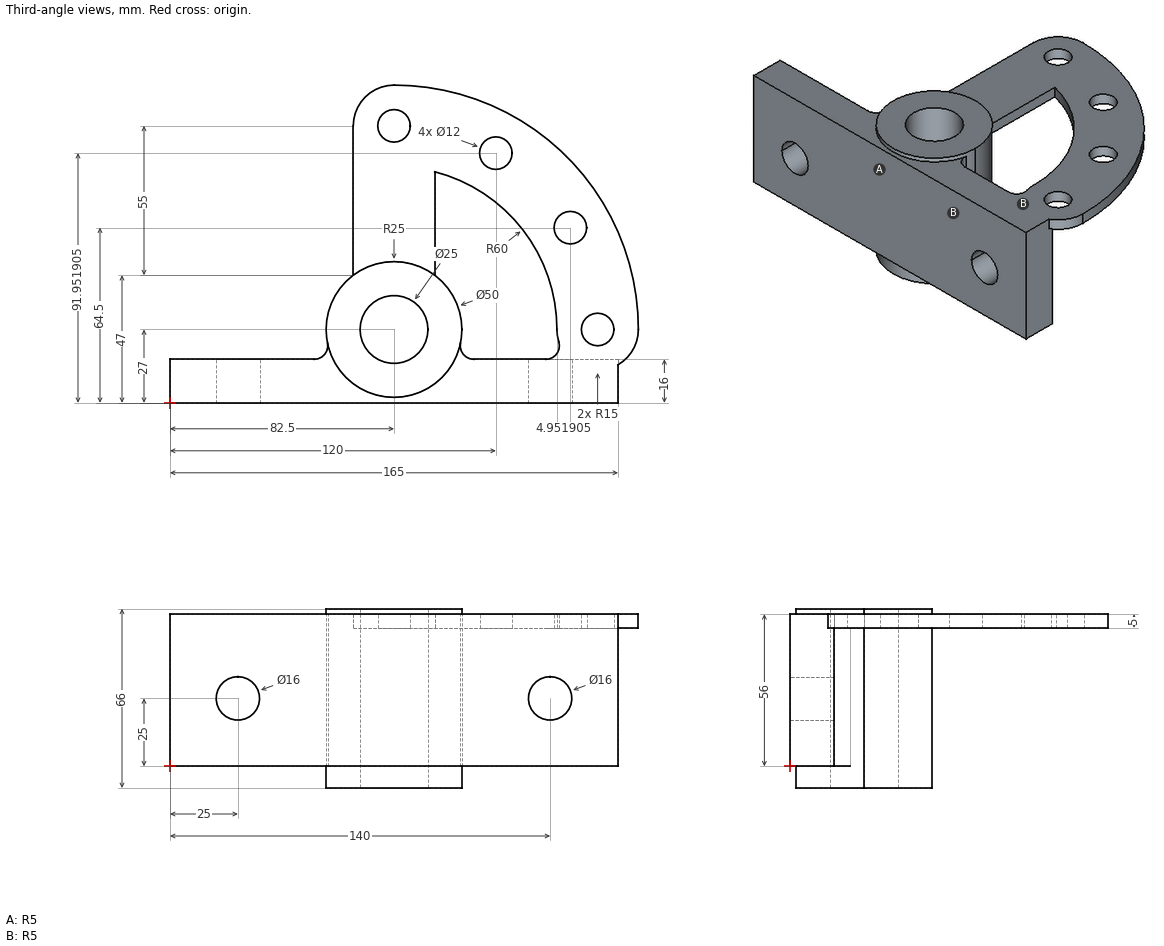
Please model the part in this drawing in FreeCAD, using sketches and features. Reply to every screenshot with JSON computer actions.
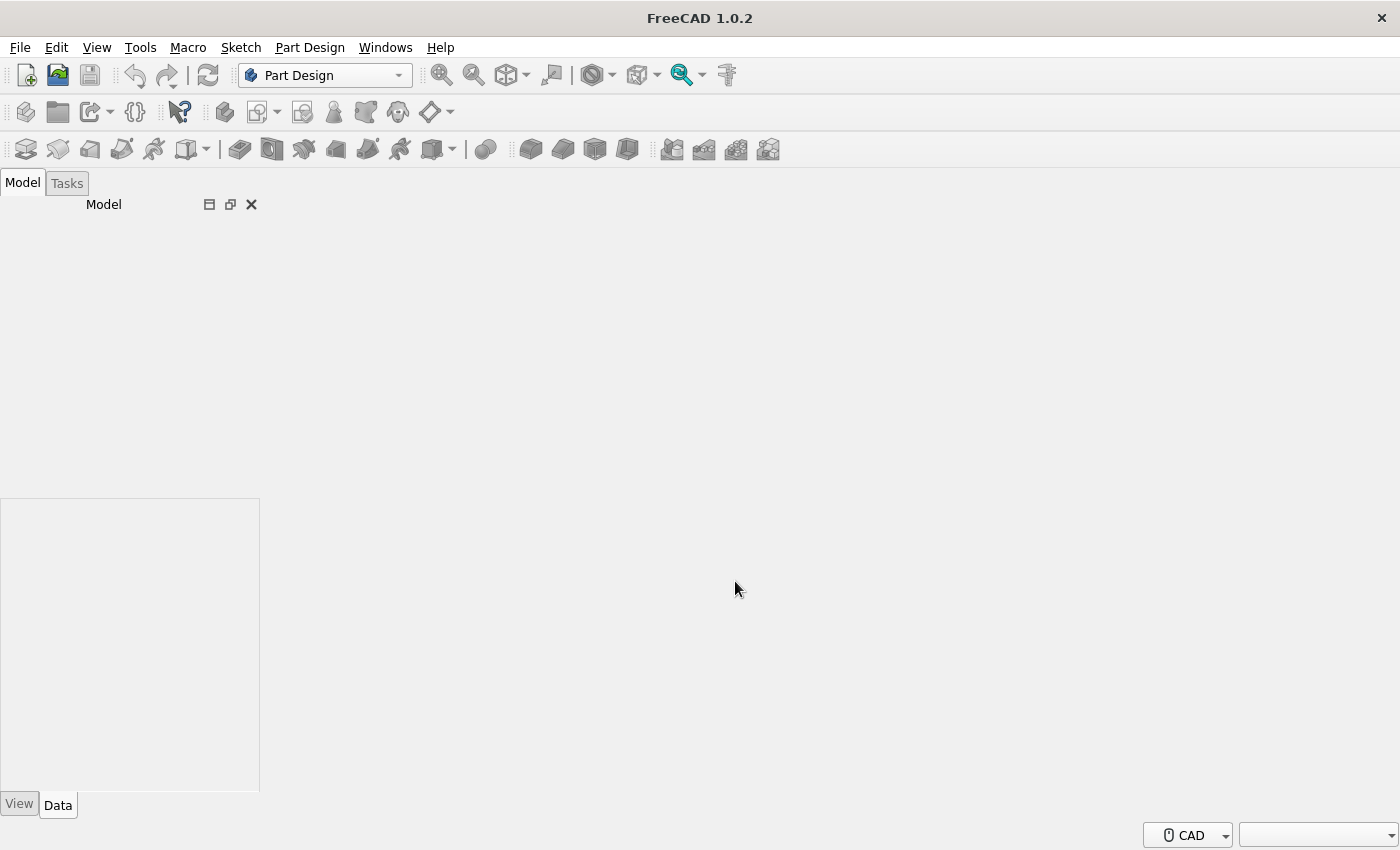
{"action": "left_click", "coordinate": [26, 76]}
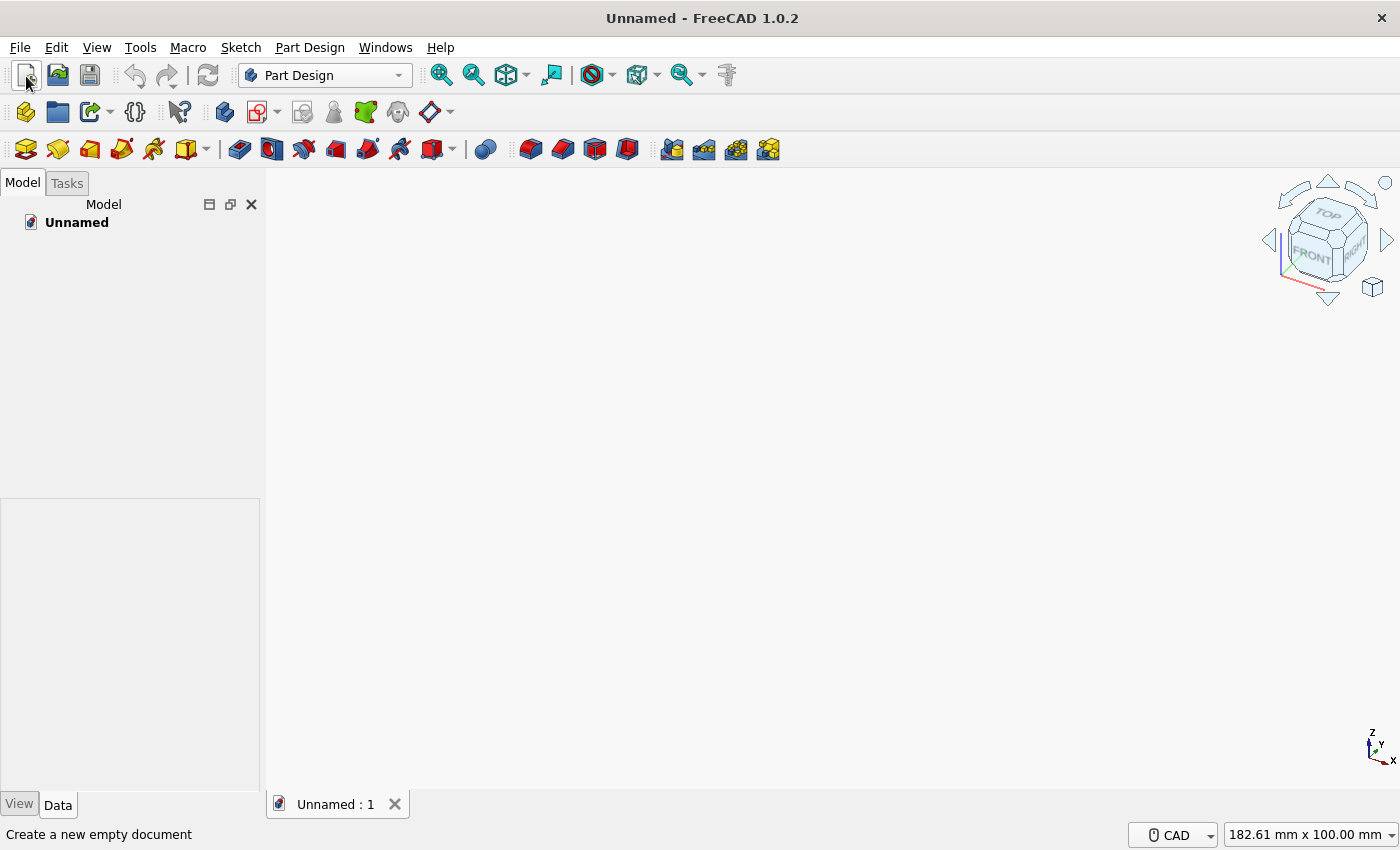
{"action": "left_click", "coordinate": [258, 112]}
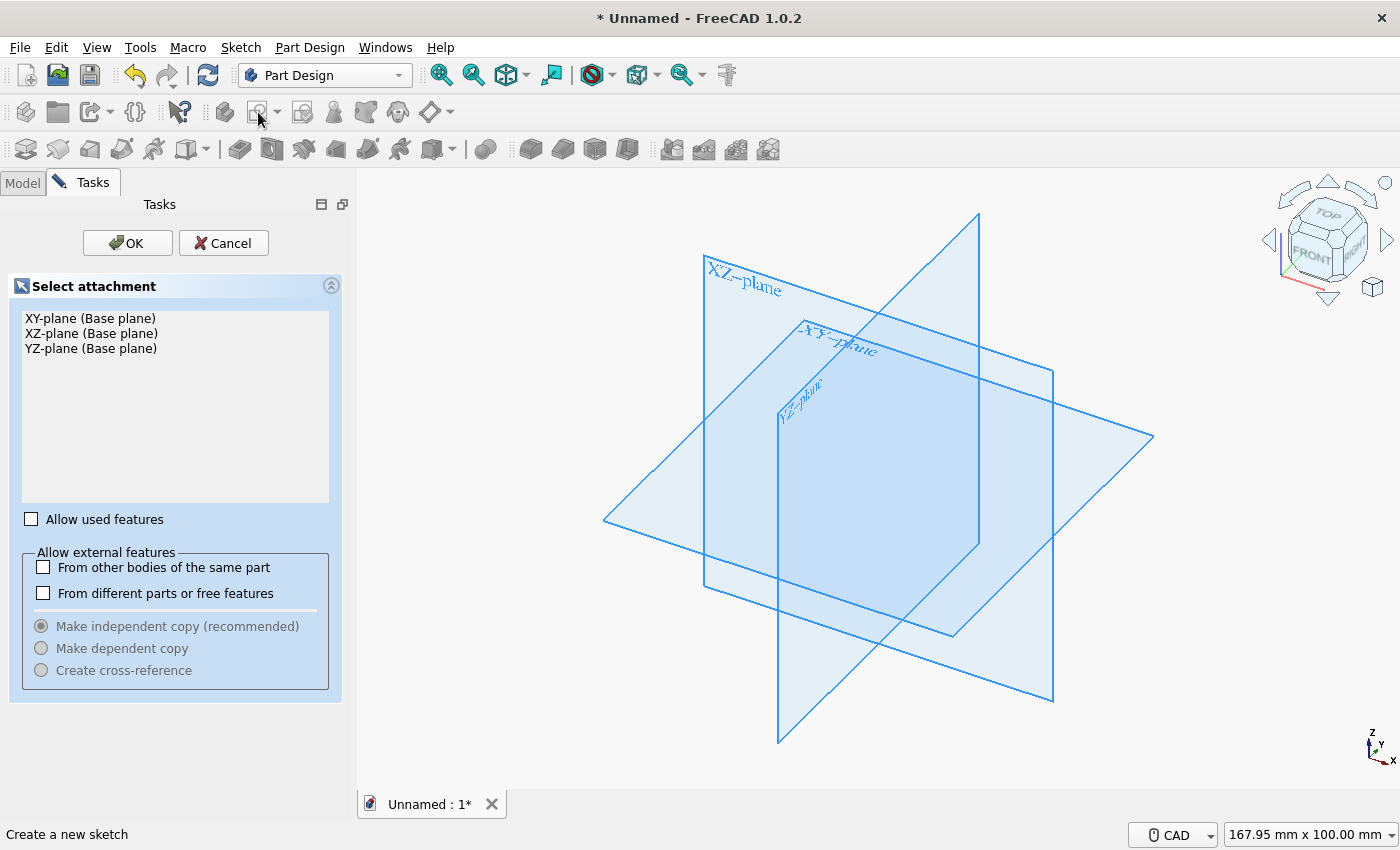
{"action": "left_click", "coordinate": [82, 318]}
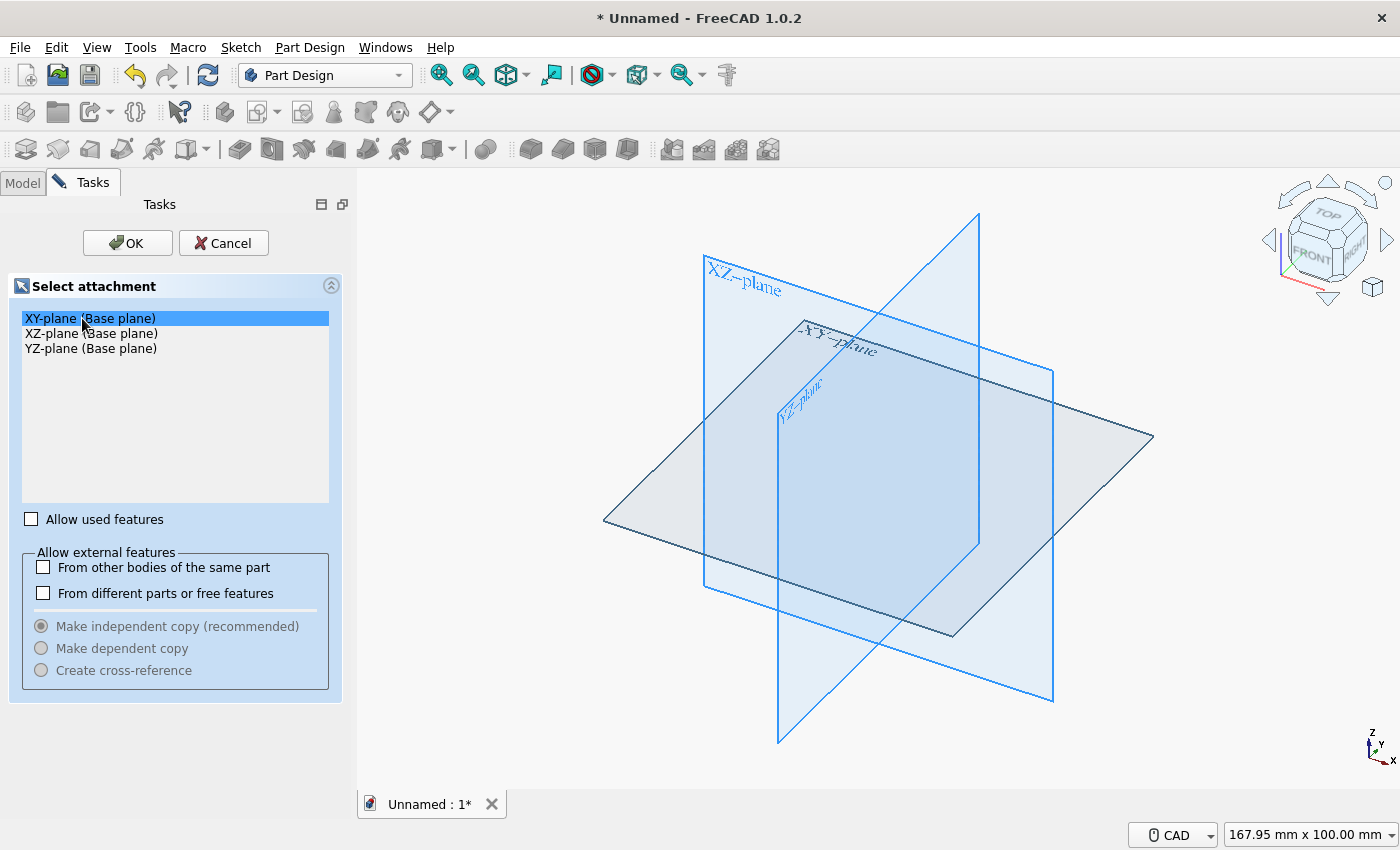
{"action": "left_click", "coordinate": [128, 243]}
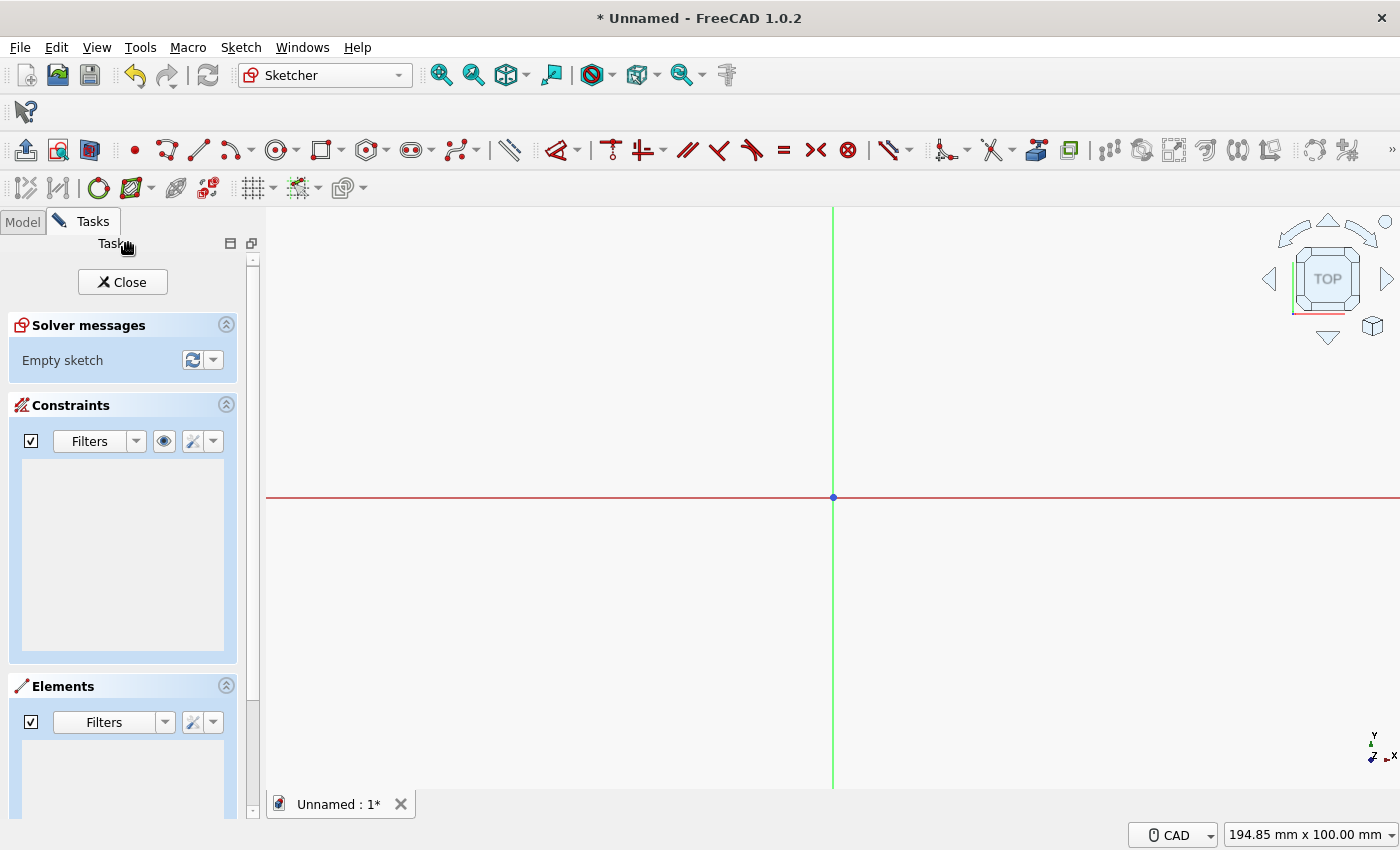
{"action": "scroll", "coordinate": [294, 555], "scroll_direction": "down", "scroll_amount": 3}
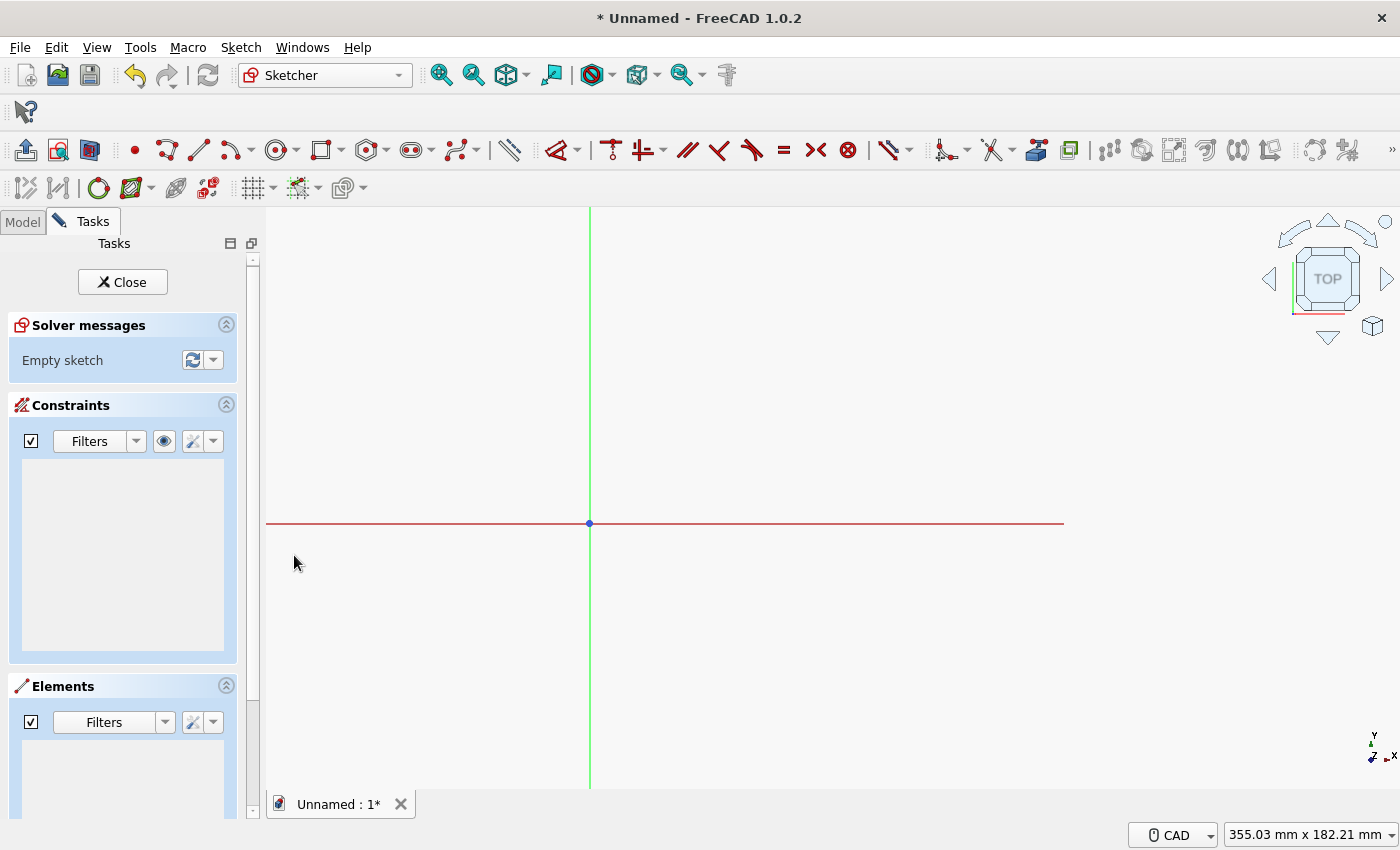
{"action": "left_click", "coordinate": [322, 150]}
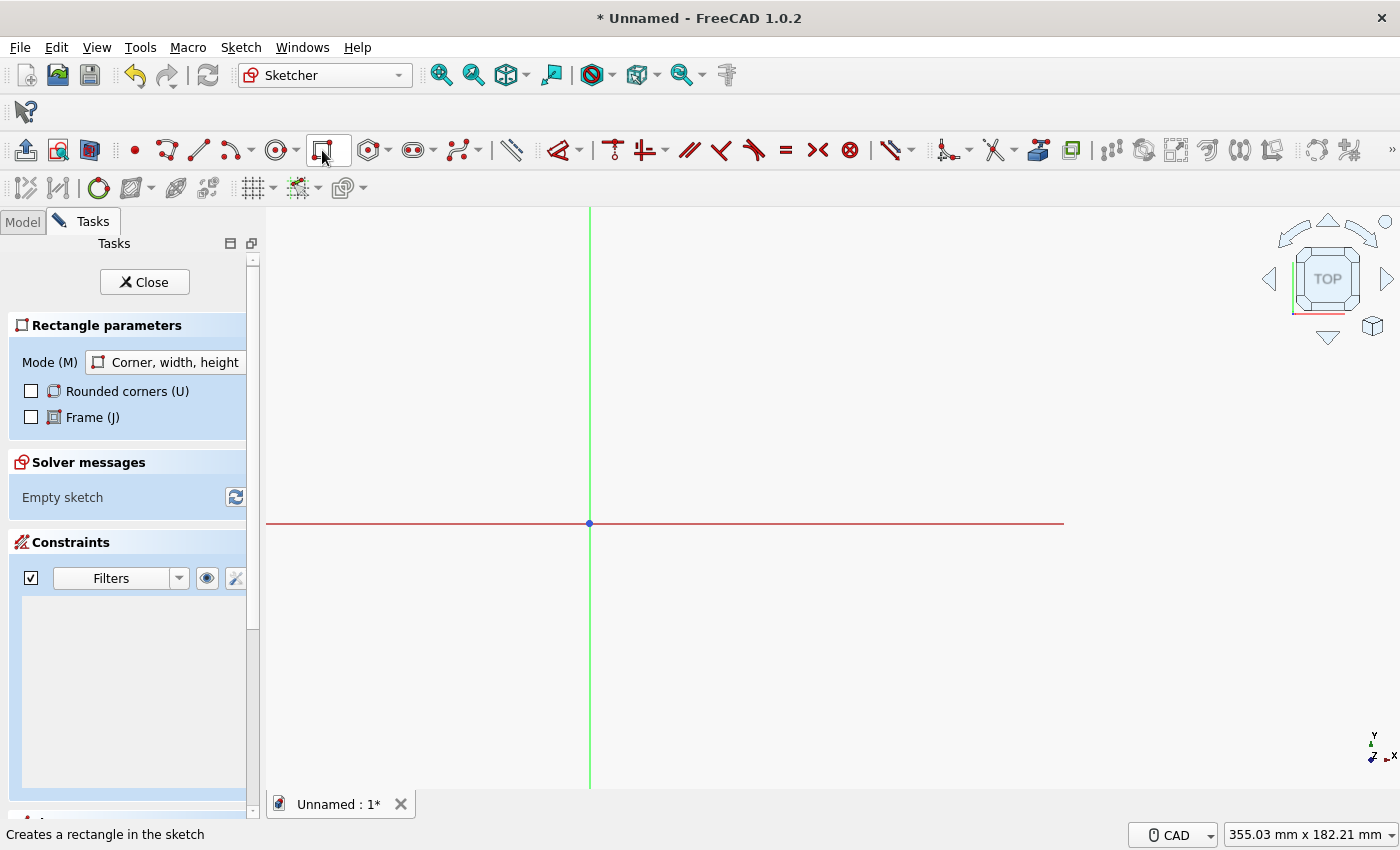
{"action": "left_click", "coordinate": [590, 524]}
{"action": "left_click", "coordinate": [1117, 473]}
{"action": "key", "text": "Escape"}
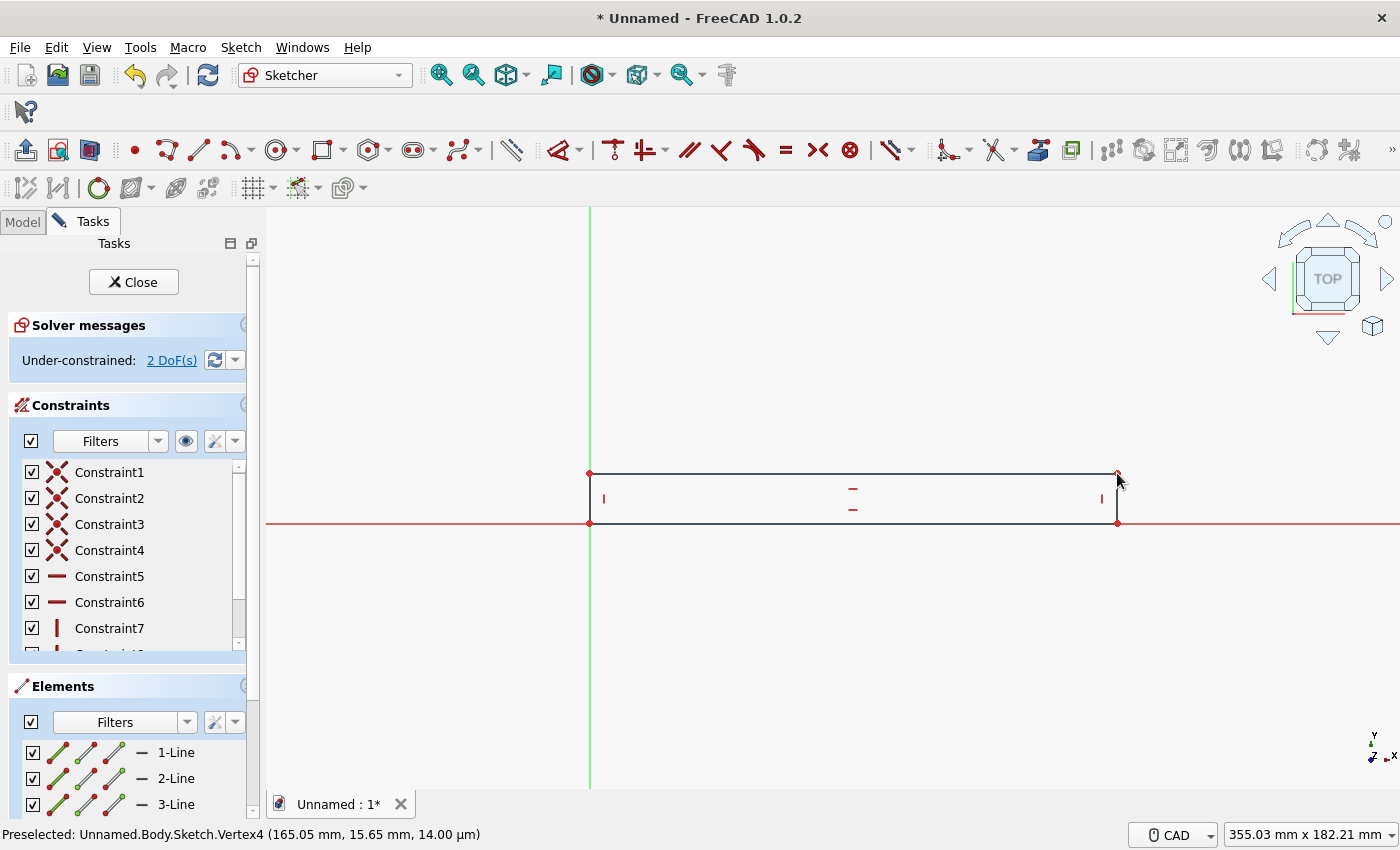
{"action": "left_click", "coordinate": [558, 150]}